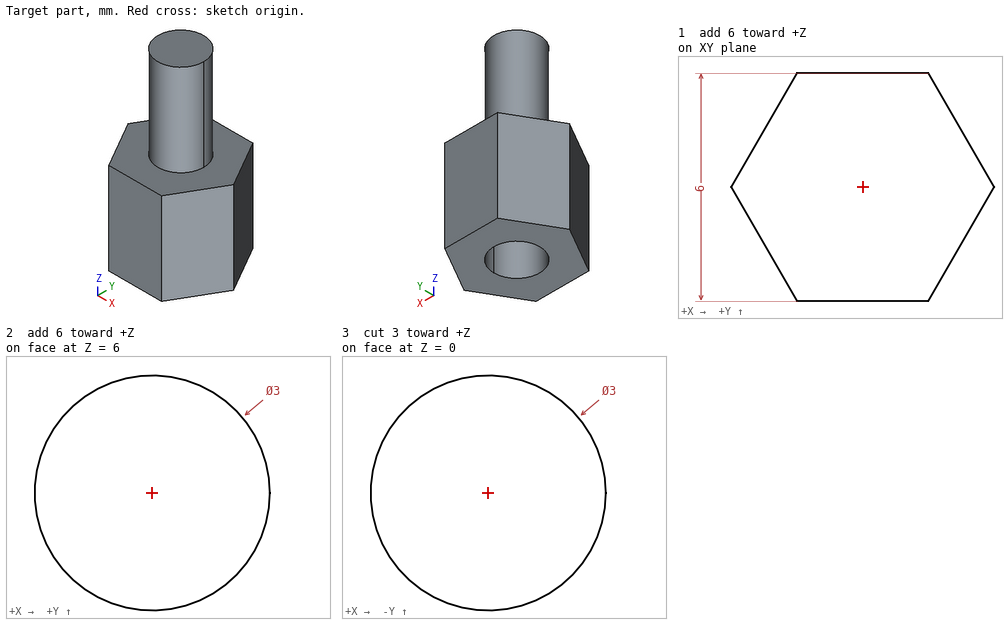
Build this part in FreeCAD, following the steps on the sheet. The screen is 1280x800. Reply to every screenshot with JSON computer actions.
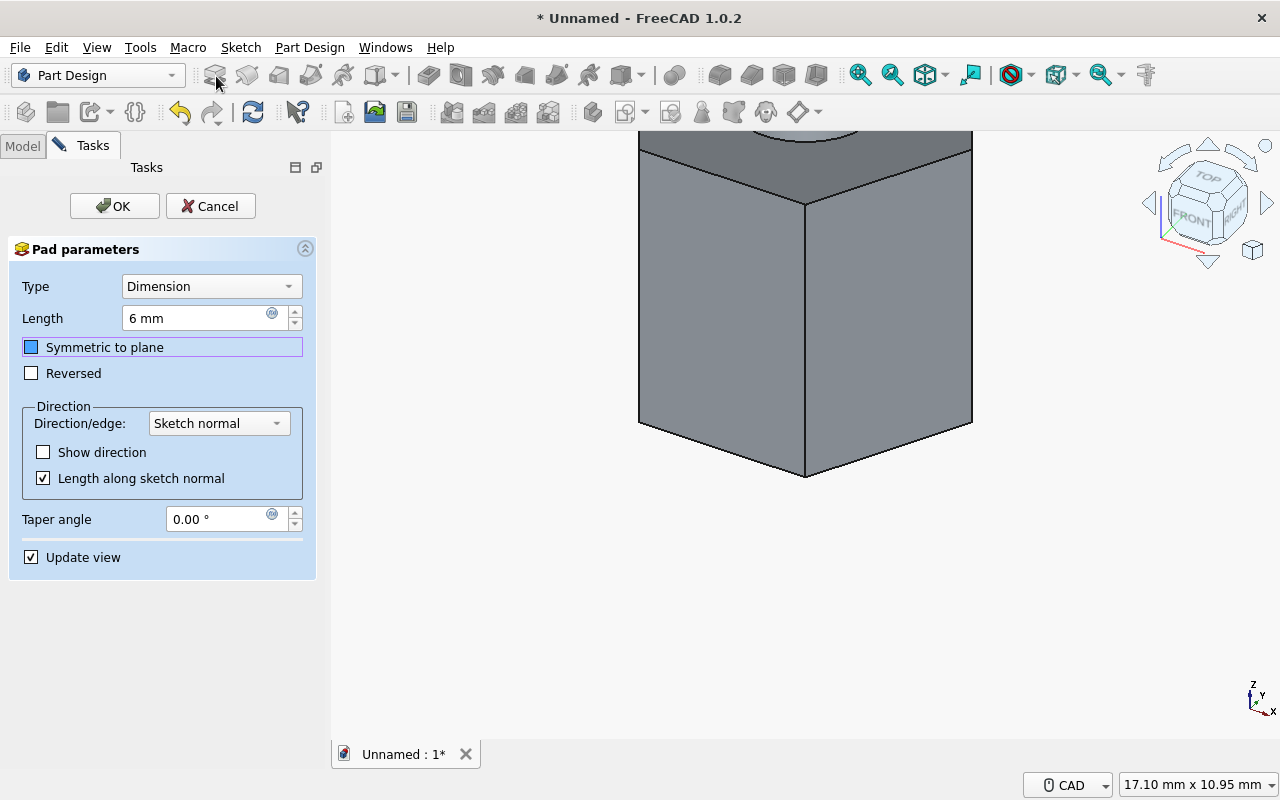
{"action": "left_click", "coordinate": [115, 206]}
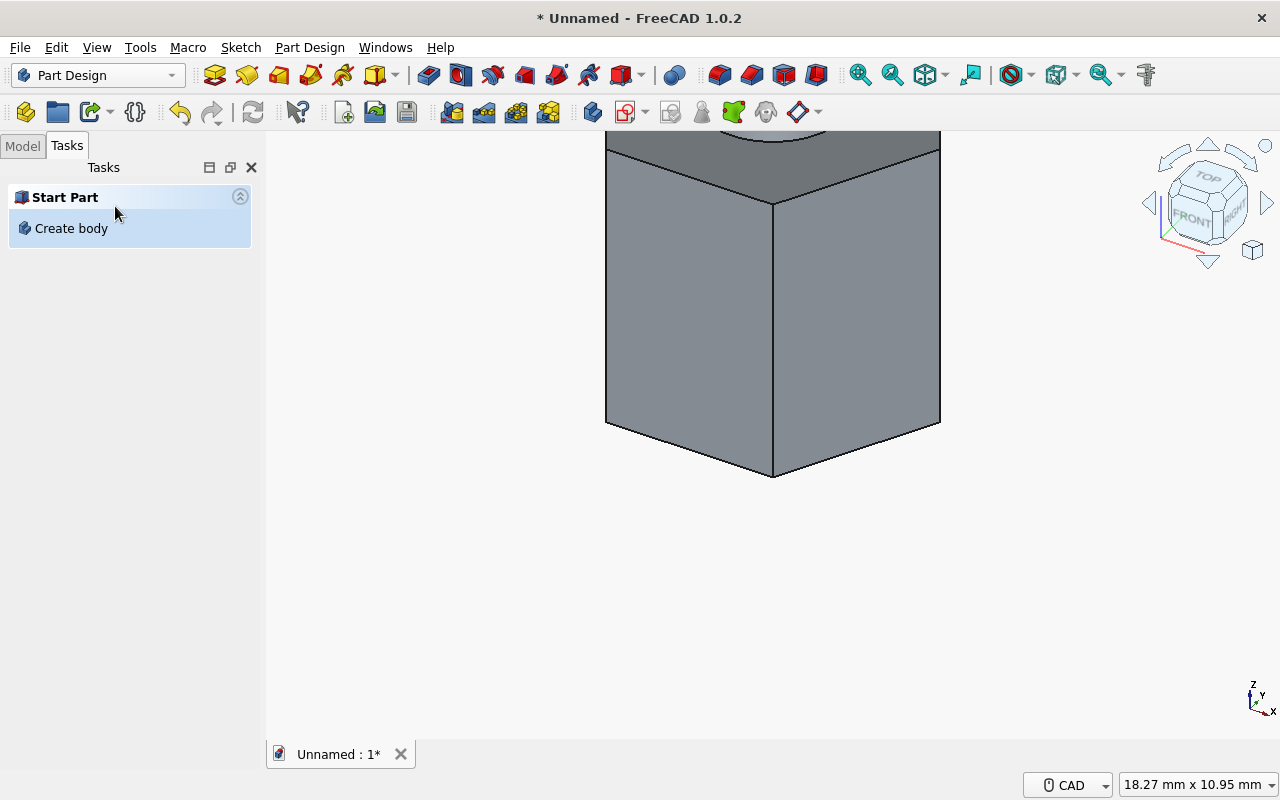
{"action": "left_click", "coordinate": [862, 76]}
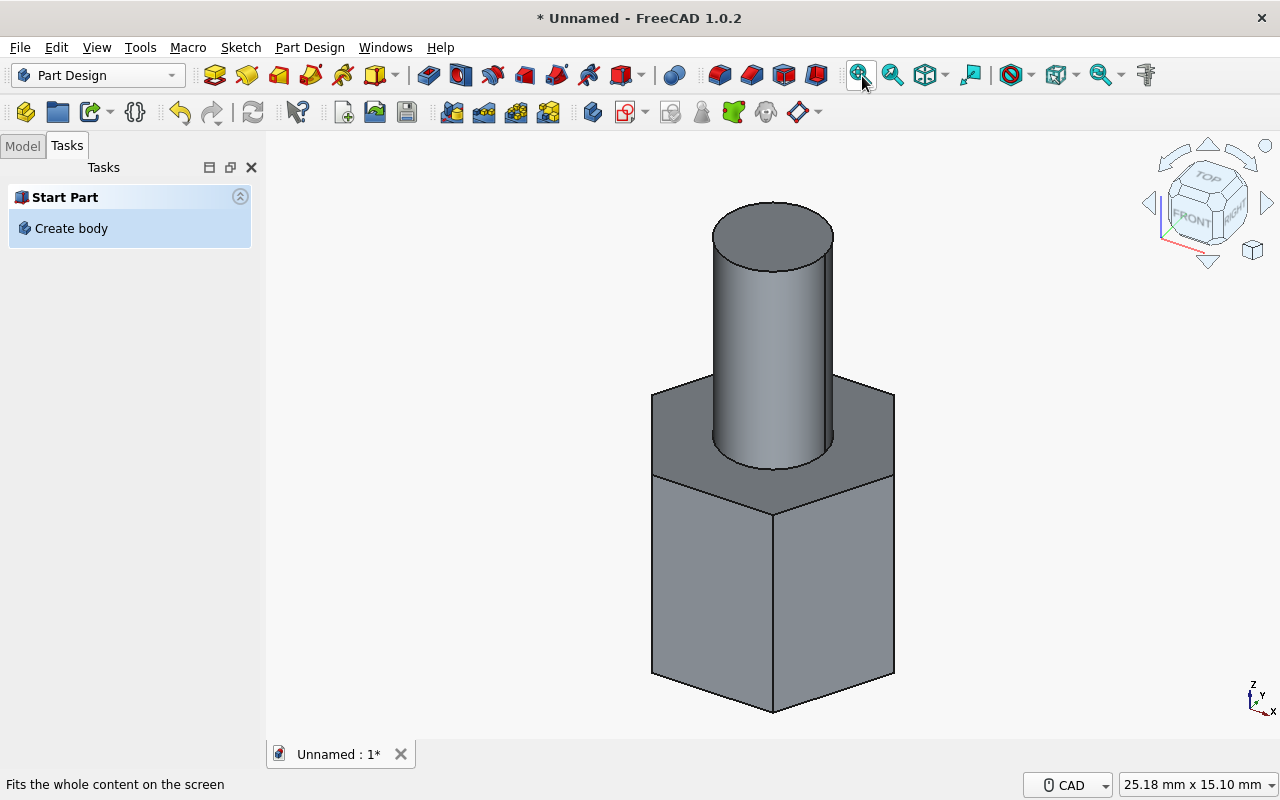
{"action": "key", "text": "5"}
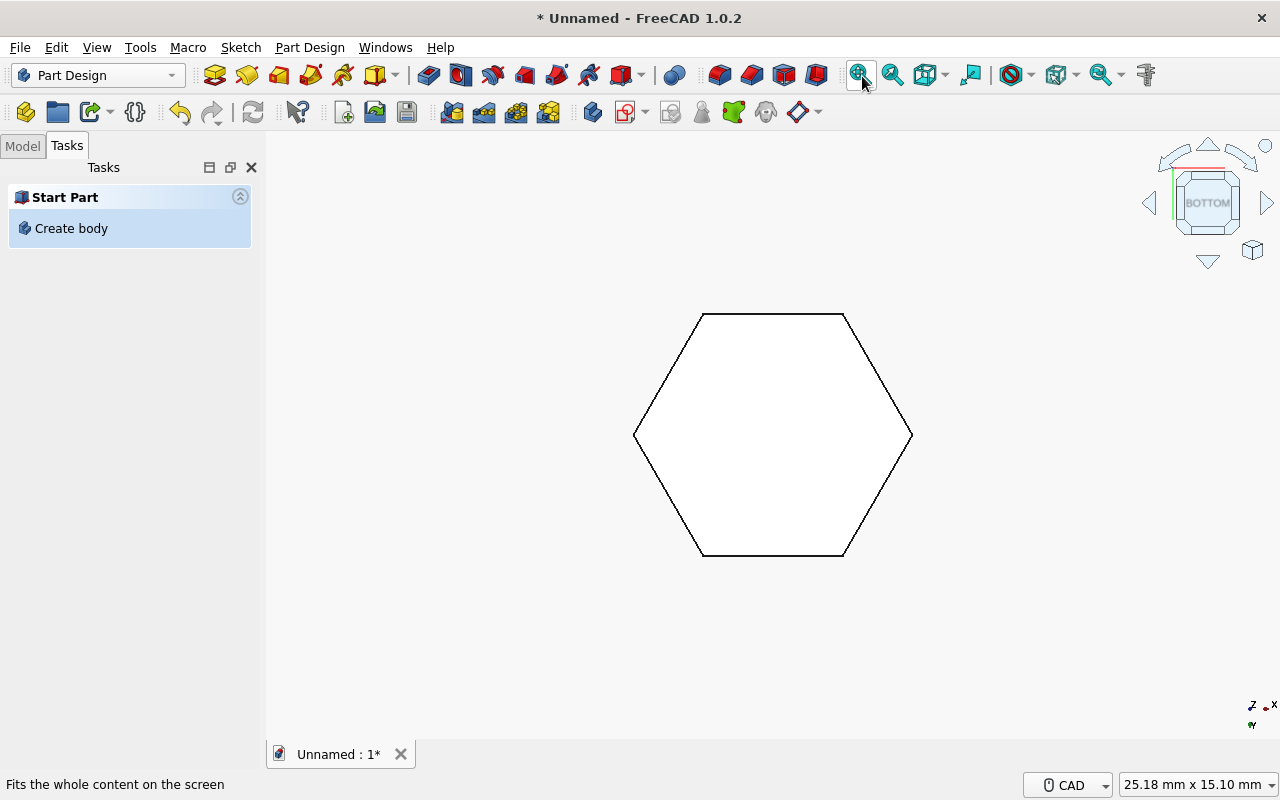
{"action": "left_click", "coordinate": [862, 76]}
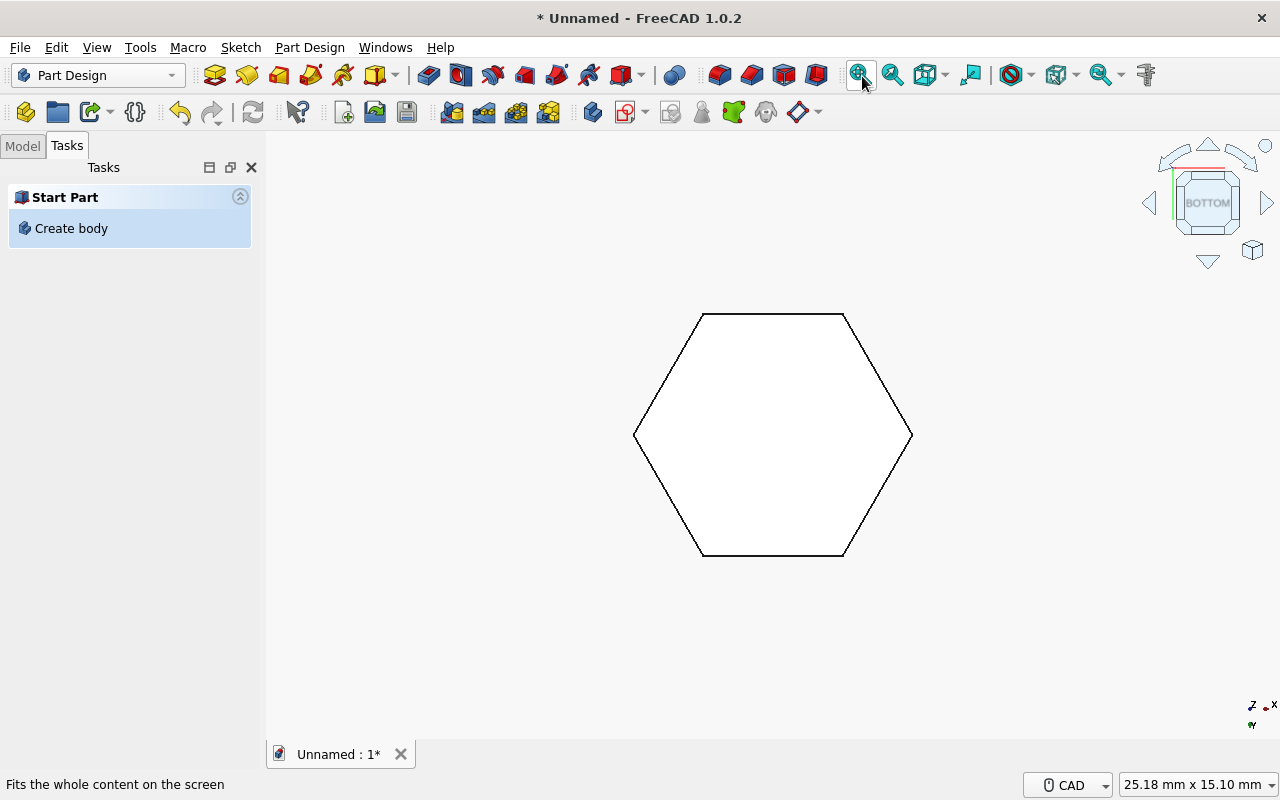
{"action": "left_click", "coordinate": [773, 434]}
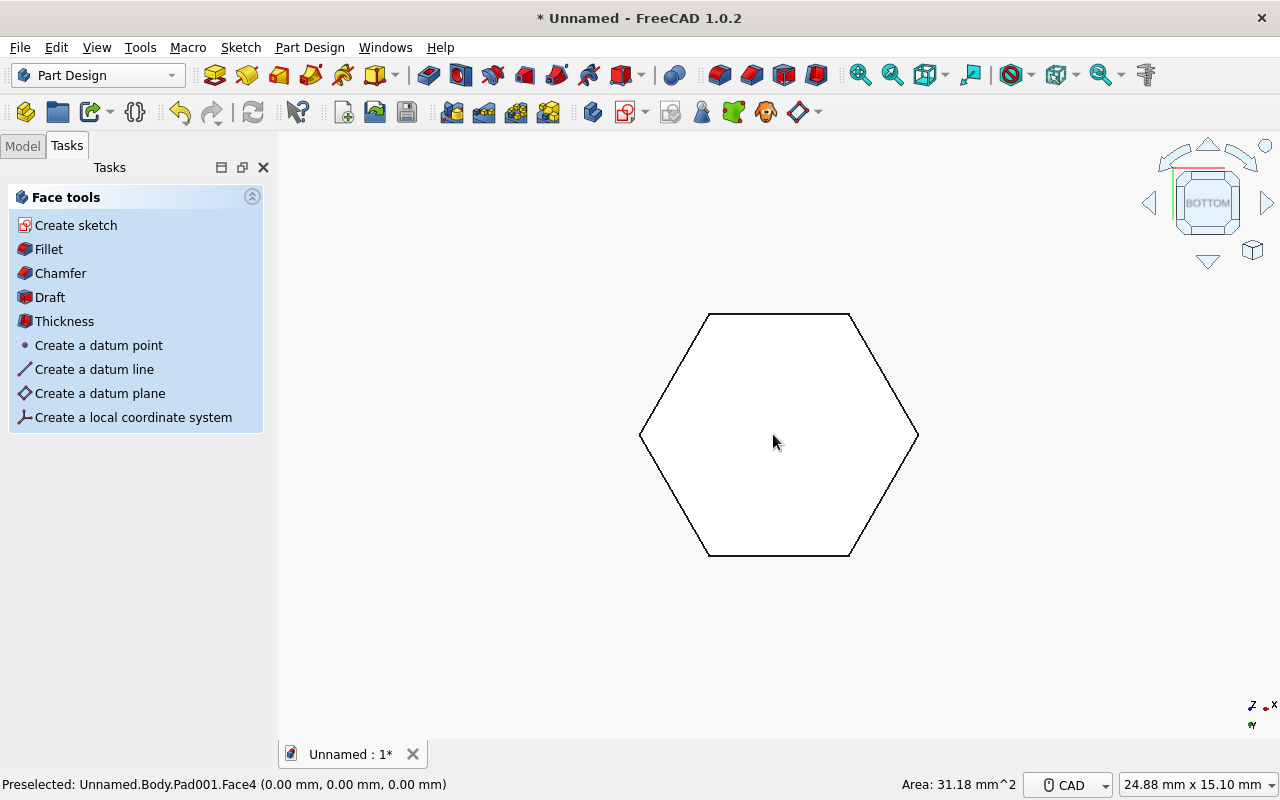
{"action": "left_click", "coordinate": [626, 112]}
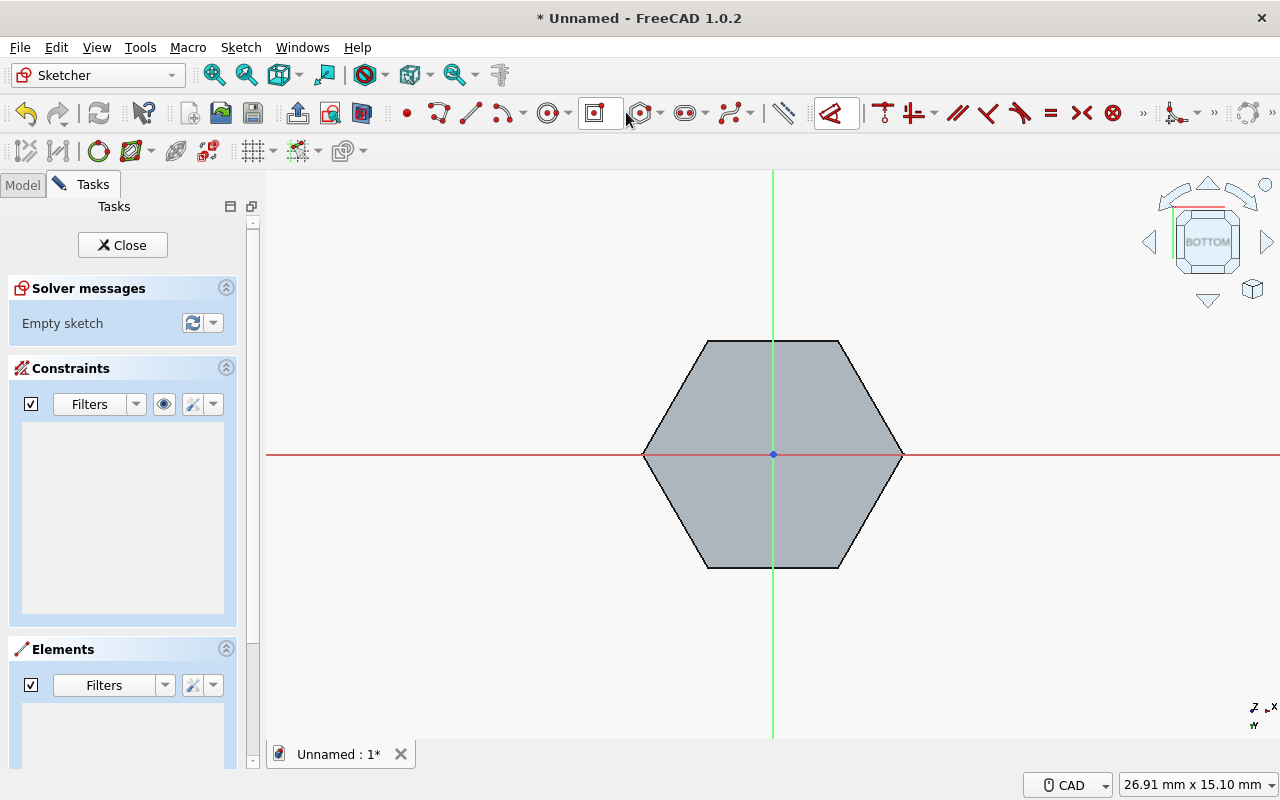
{"action": "scroll", "coordinate": [803, 455], "scroll_direction": "up", "scroll_amount": 6}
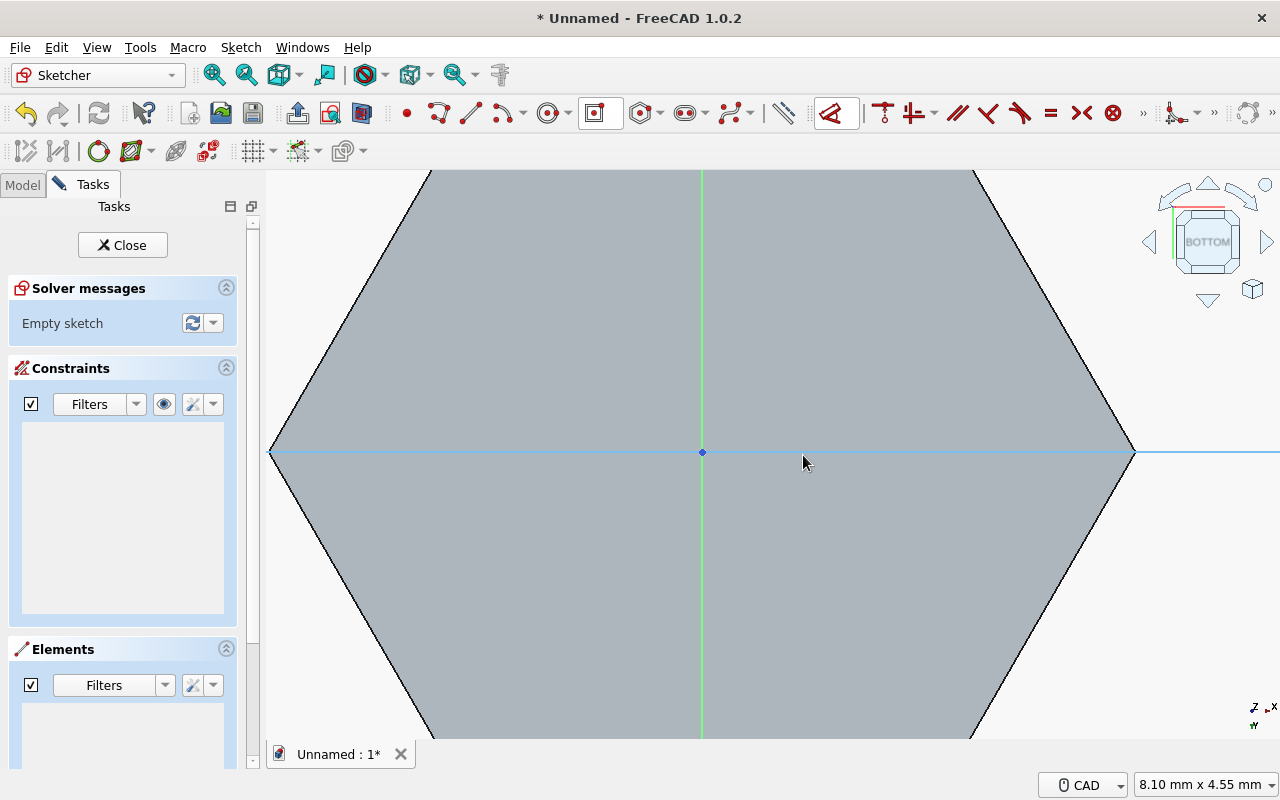
{"action": "key", "text": "g c"}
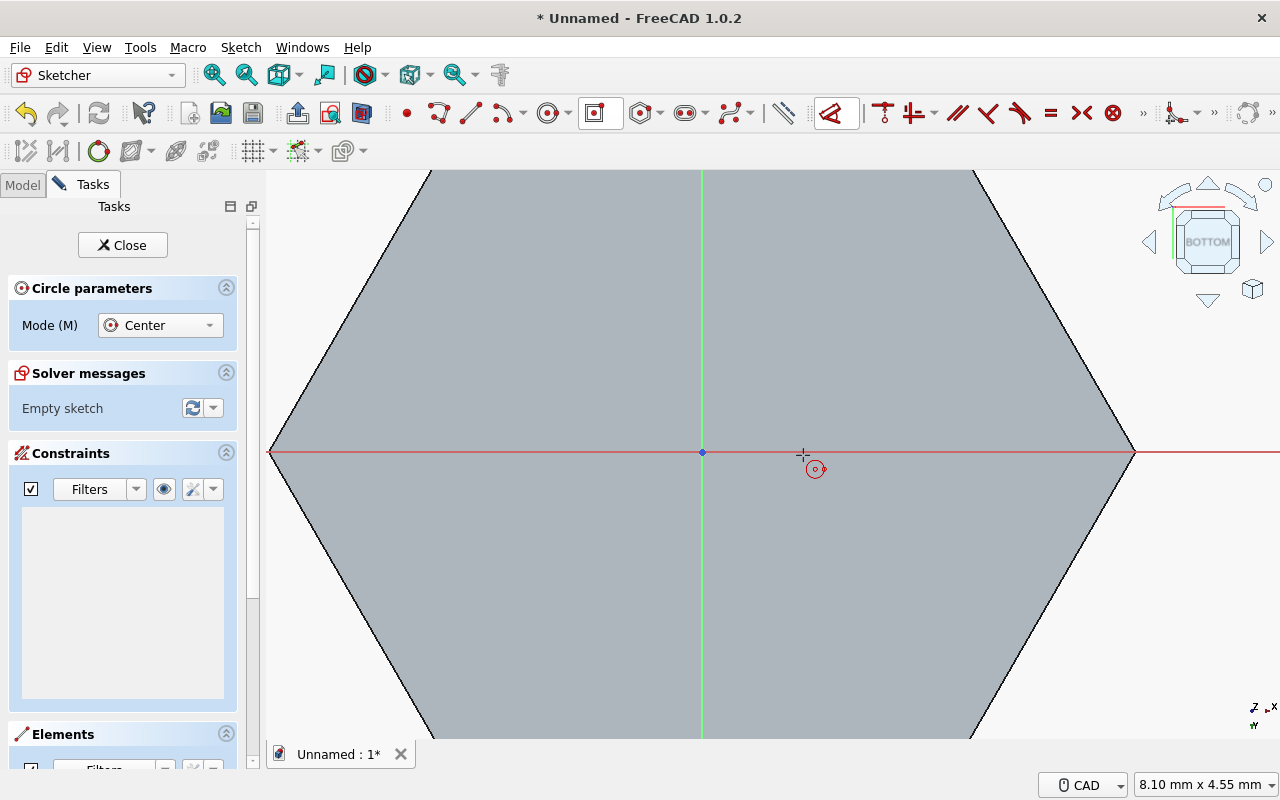
{"action": "left_click", "coordinate": [702, 452]}
{"action": "left_click", "coordinate": [835, 319]}
{"action": "key", "text": "Escape"}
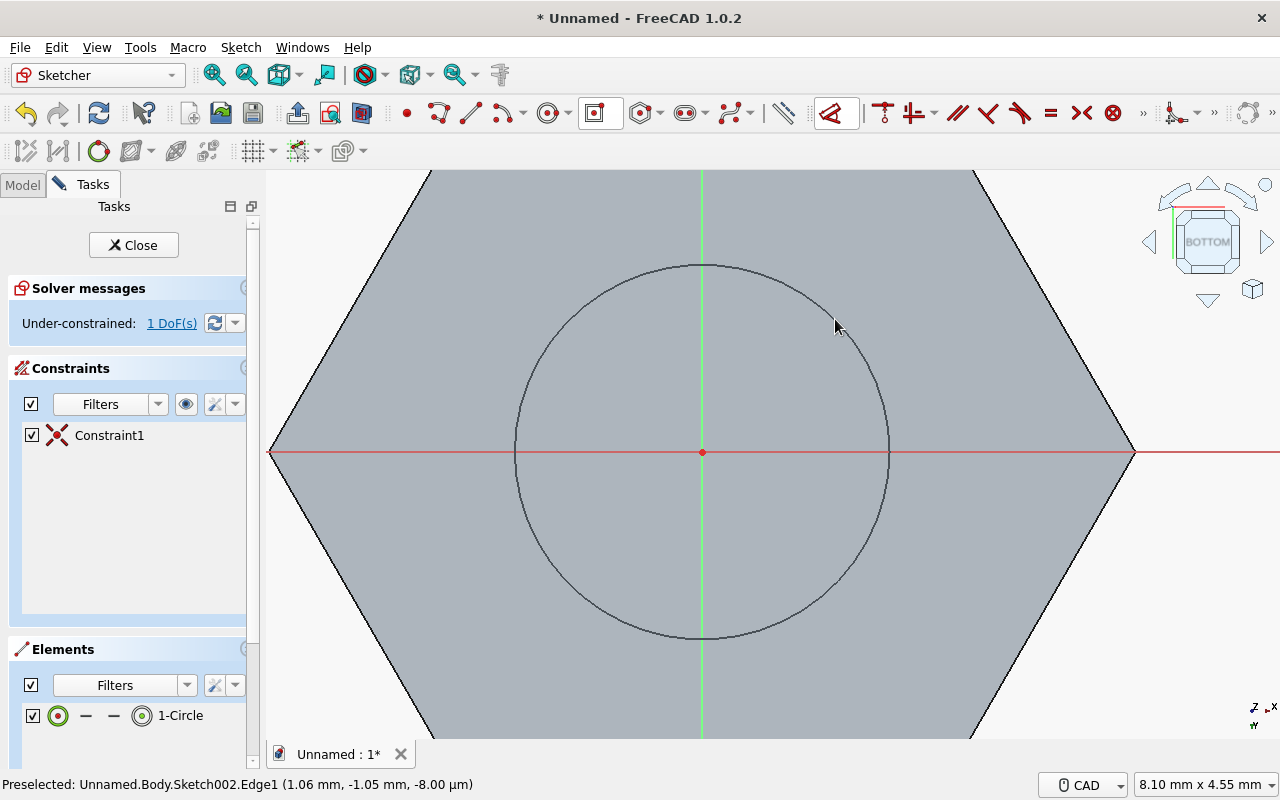
{"action": "left_click", "coordinate": [834, 319]}